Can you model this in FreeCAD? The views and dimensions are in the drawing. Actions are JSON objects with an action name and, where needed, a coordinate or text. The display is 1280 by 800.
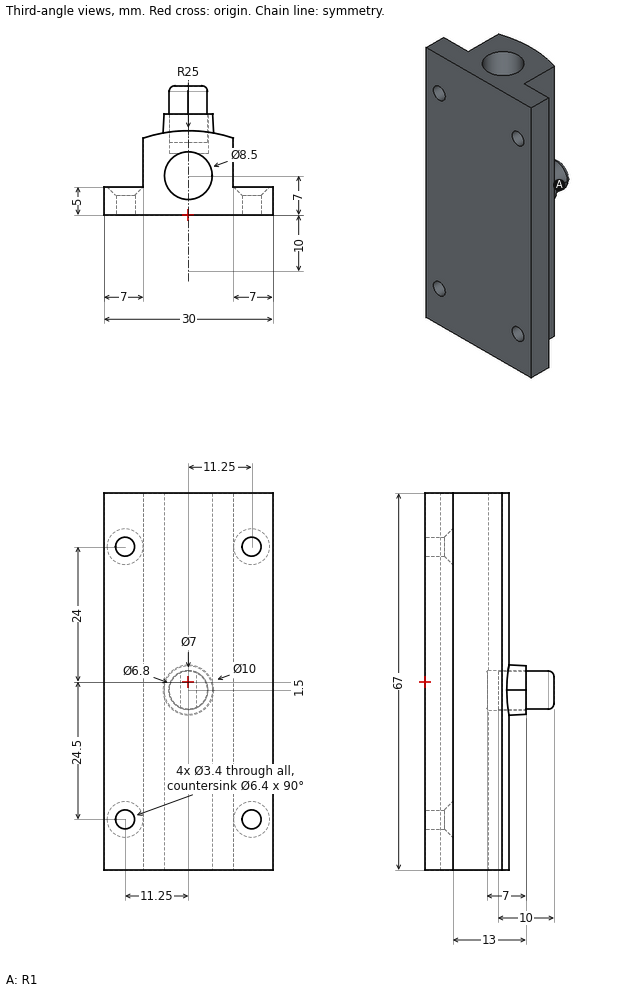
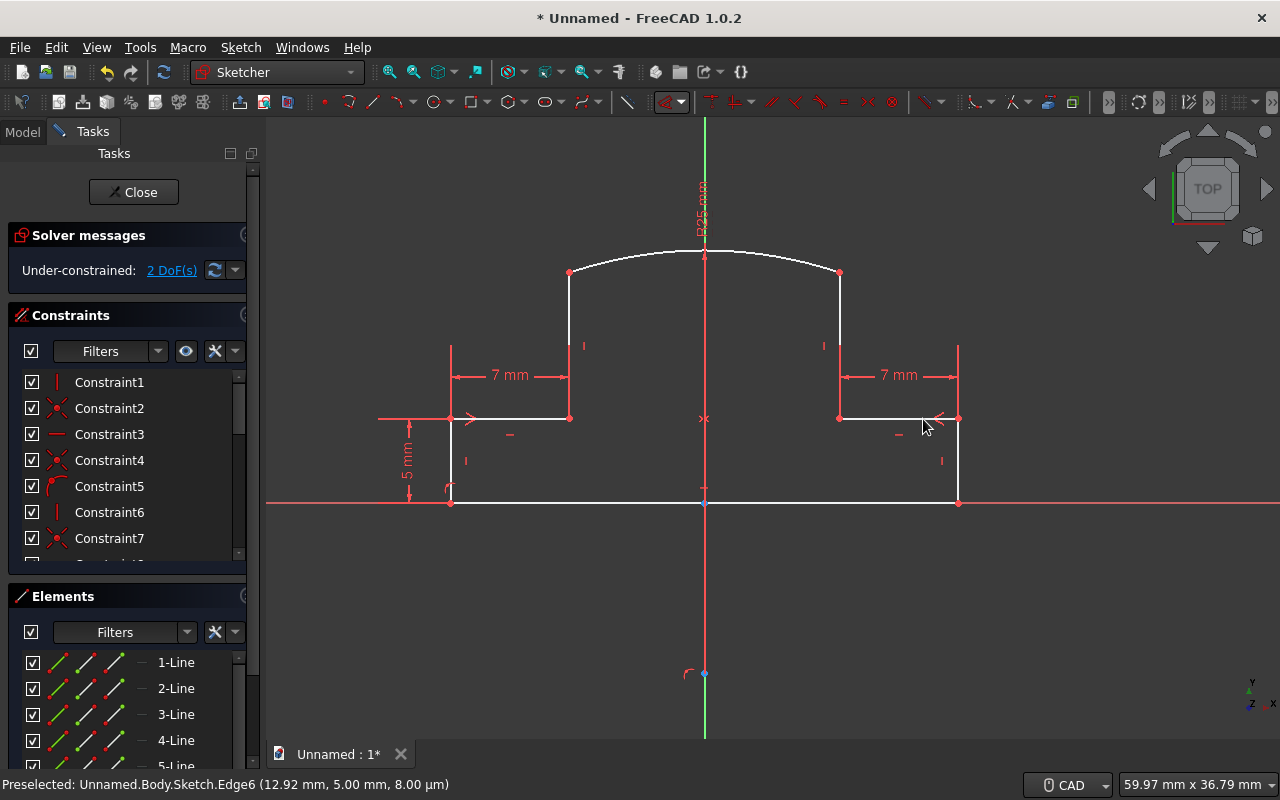
{"action": "left_click", "coordinate": [603, 503]}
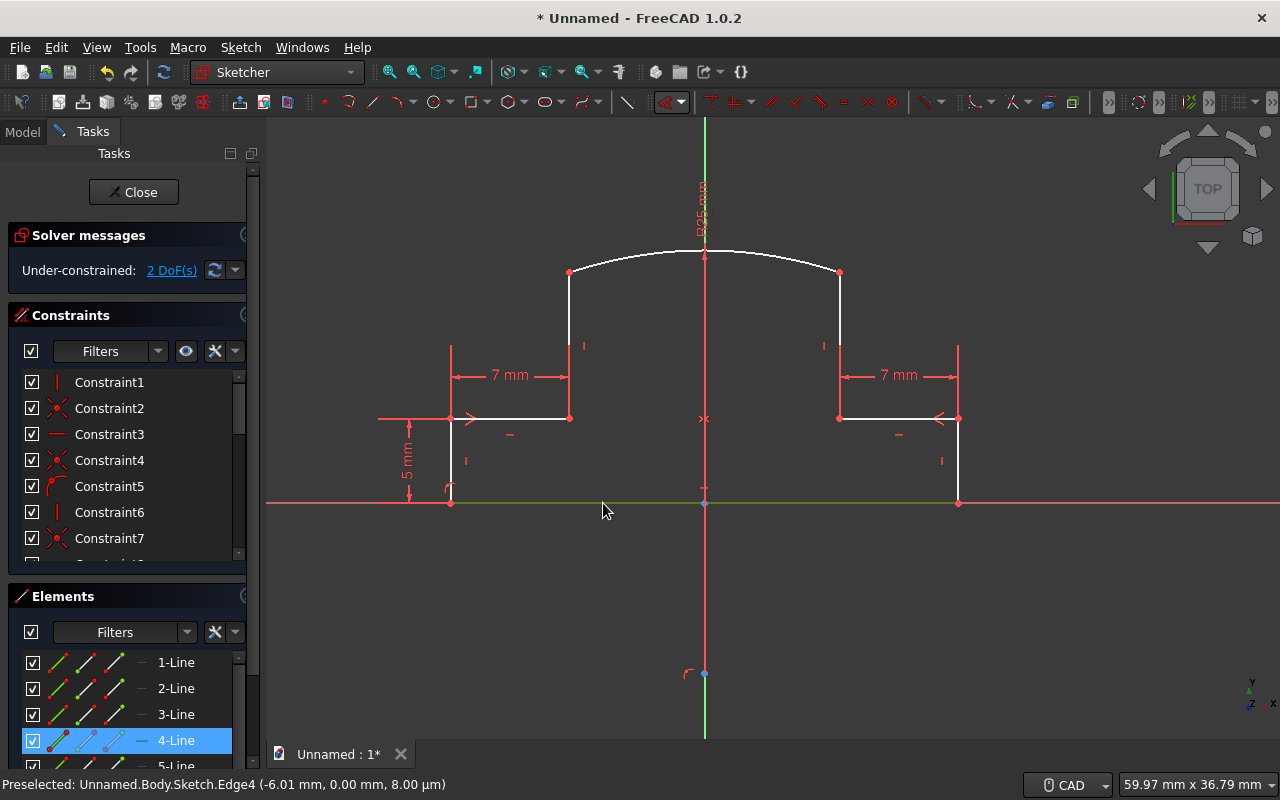
{"action": "key", "text": "l"}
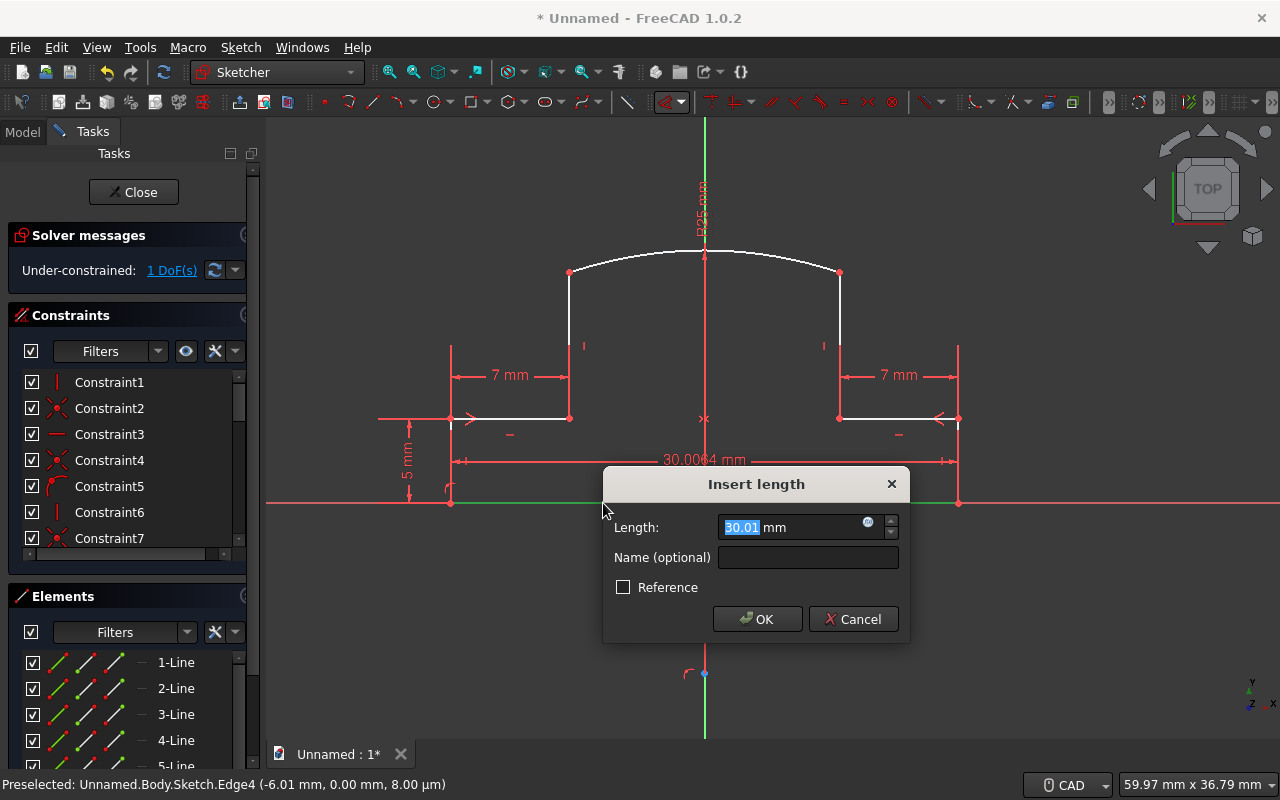
{"action": "type", "text": "30"}
{"action": "key", "text": "Return"}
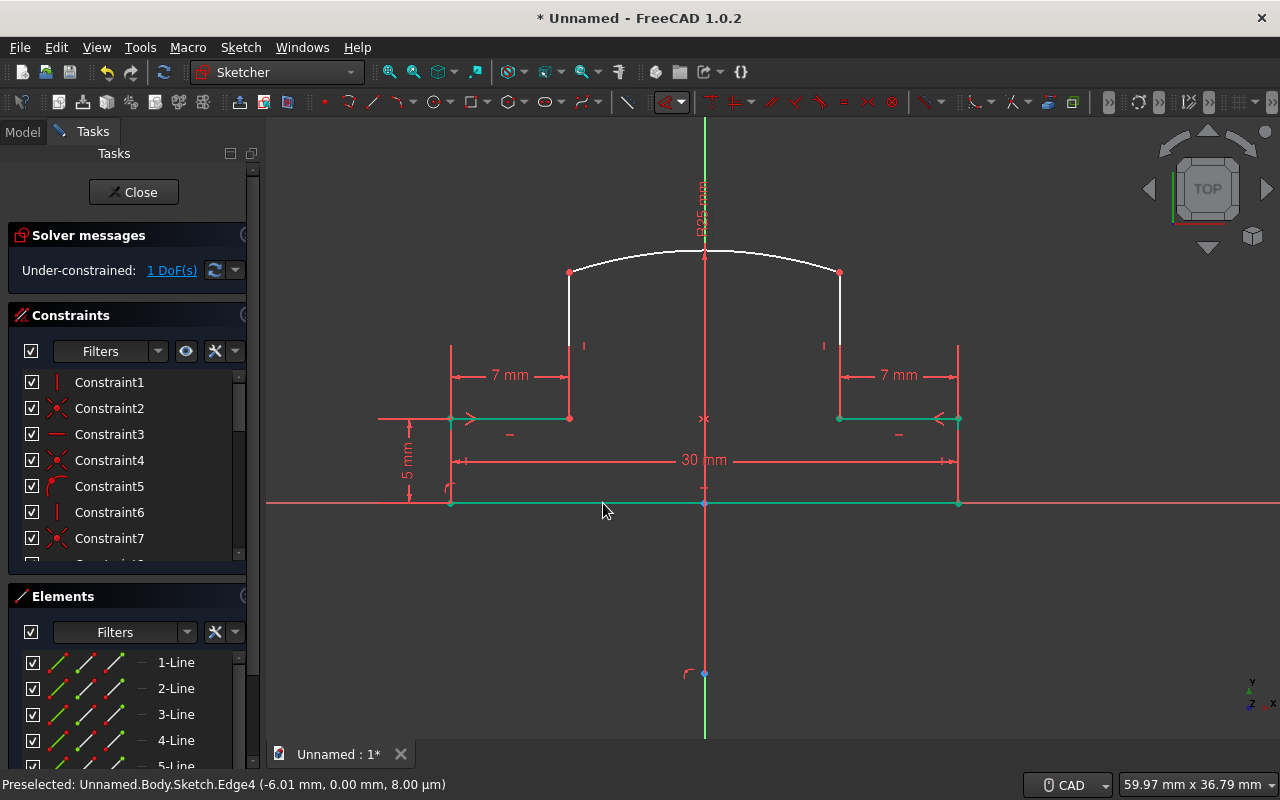
{"action": "left_click", "coordinate": [705, 673]}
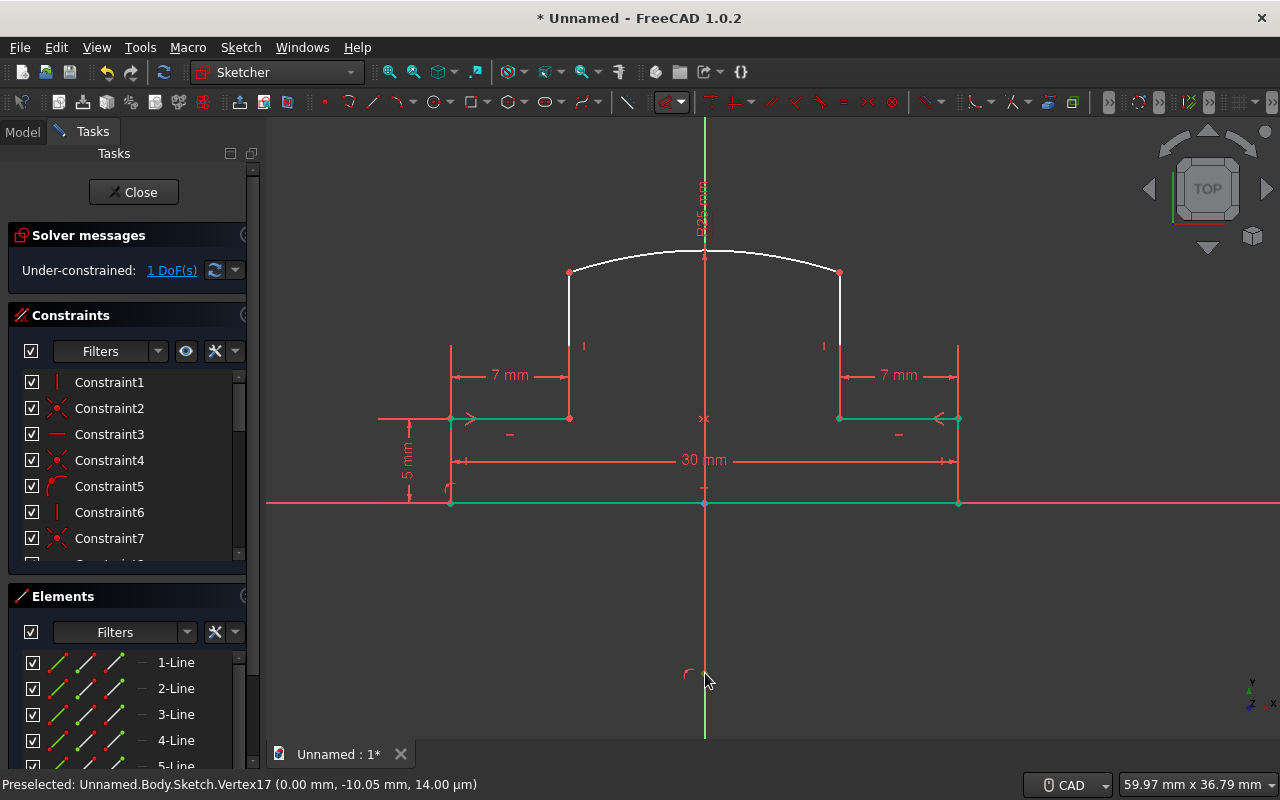
{"action": "key", "text": "i"}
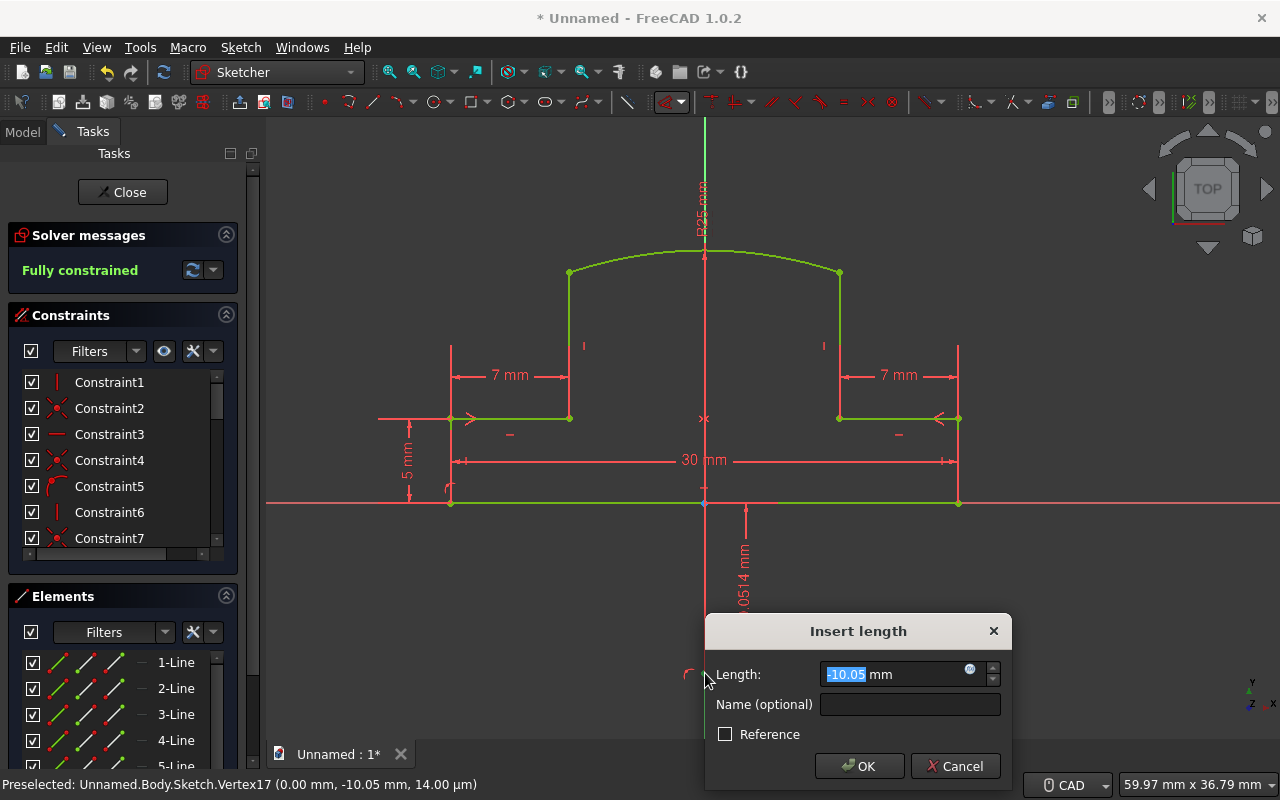
{"action": "type", "text": "-10"}
{"action": "key", "text": "Return"}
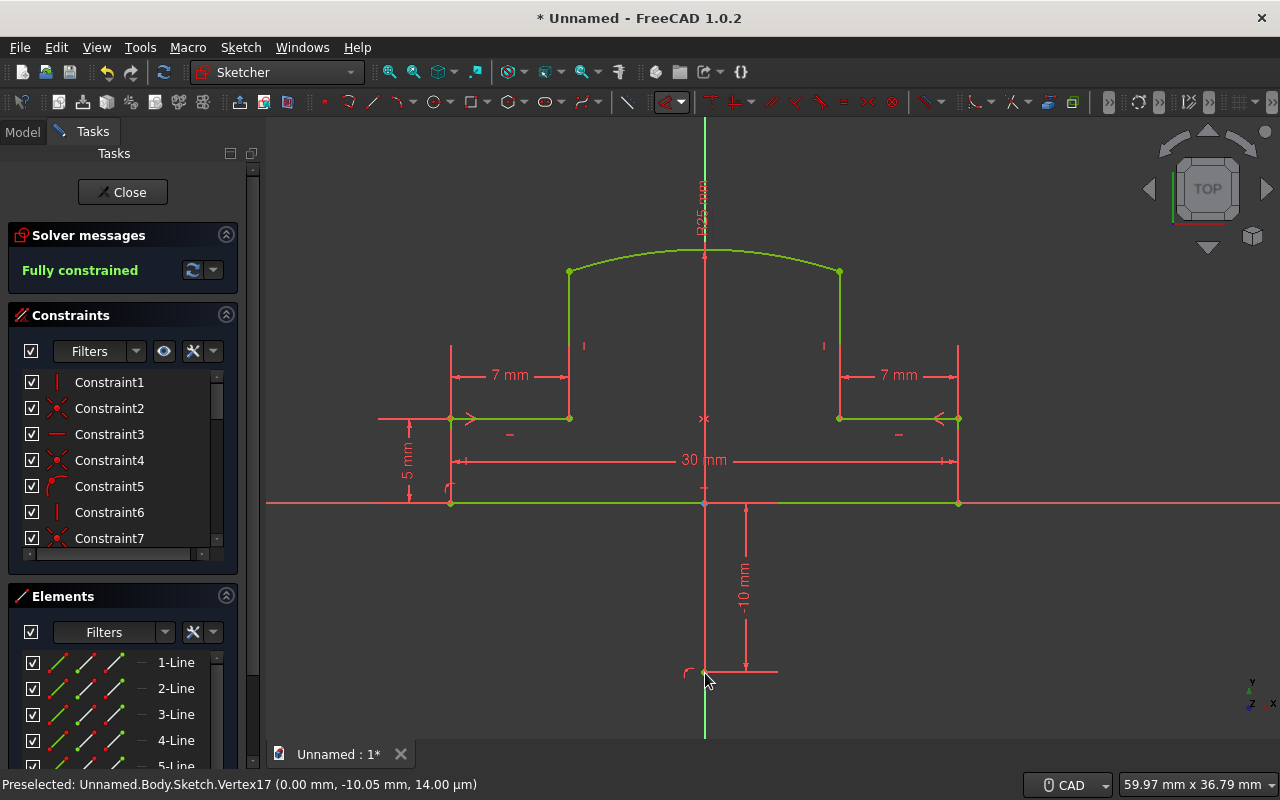
{"action": "left_click", "coordinate": [123, 192]}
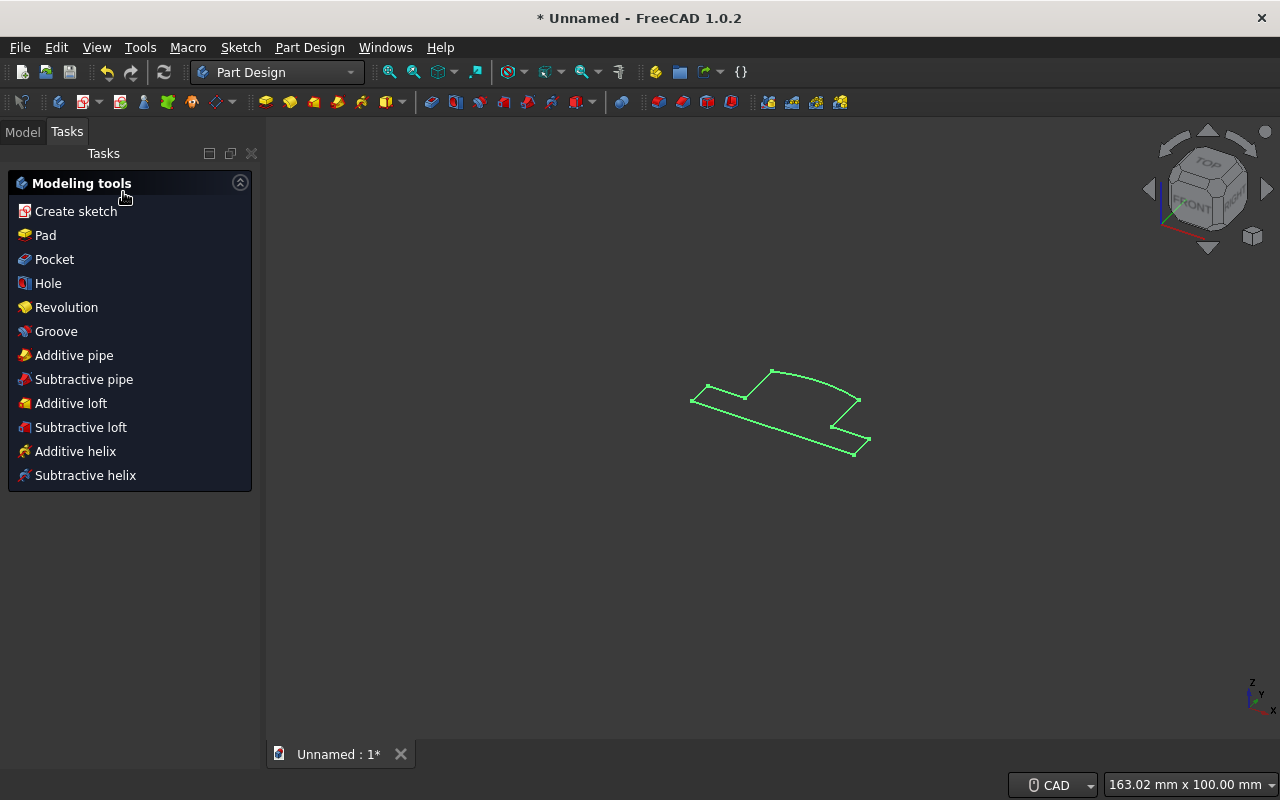
{"action": "left_click", "coordinate": [266, 102]}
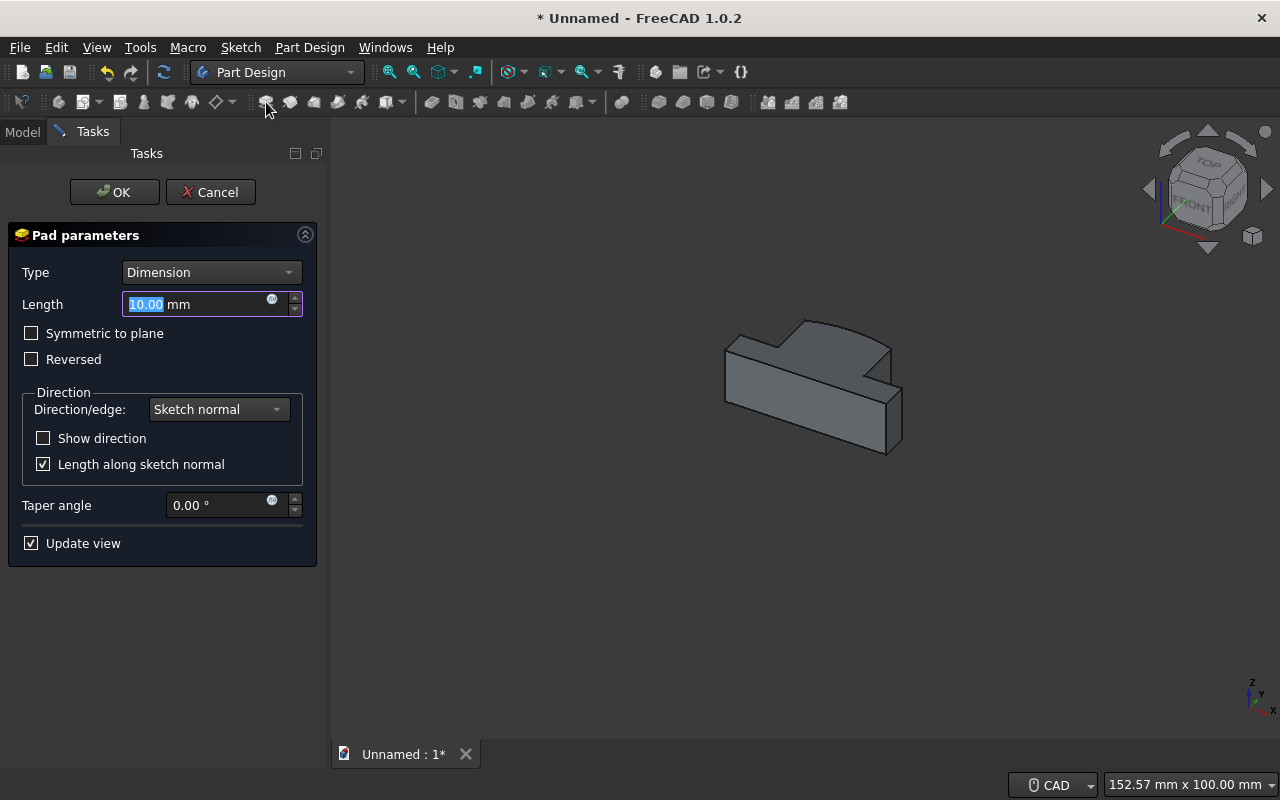
{"action": "type", "text": "67"}
{"action": "key", "text": "Tab"}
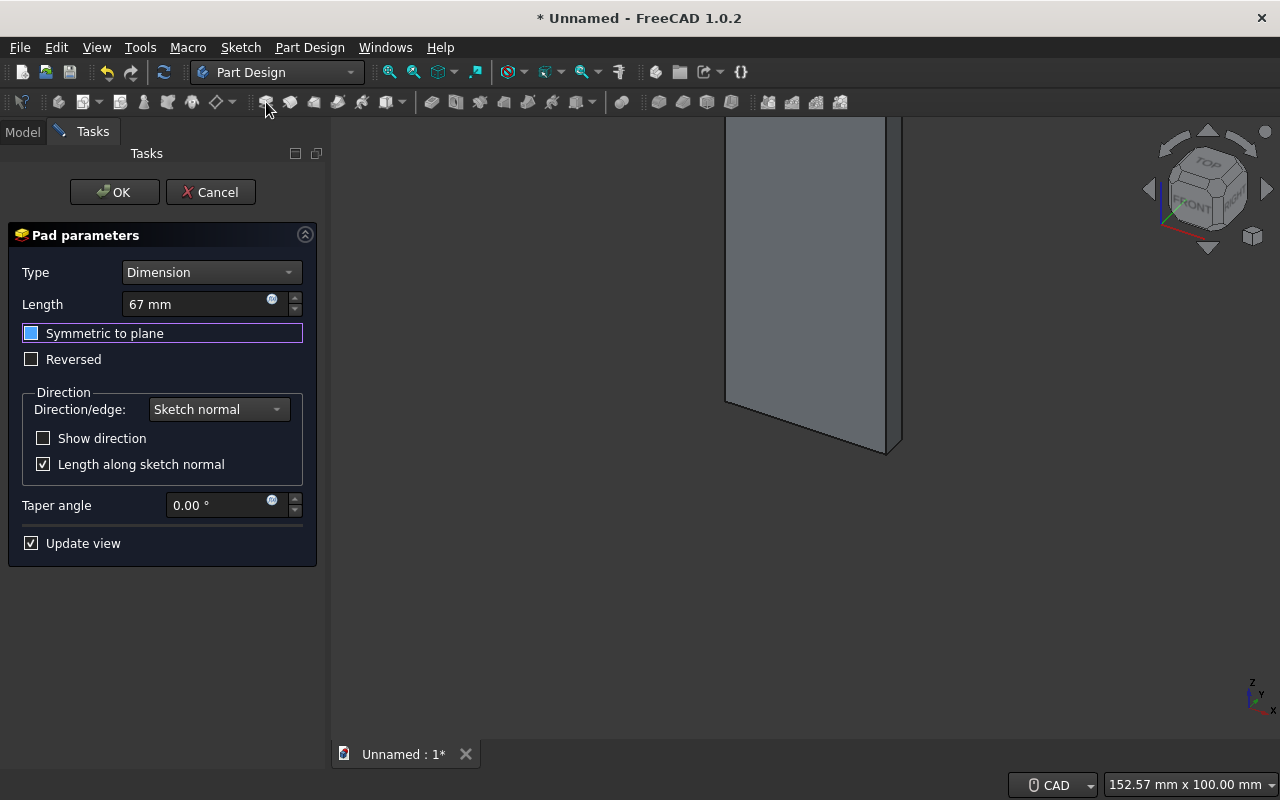
{"action": "left_click", "coordinate": [30, 333]}